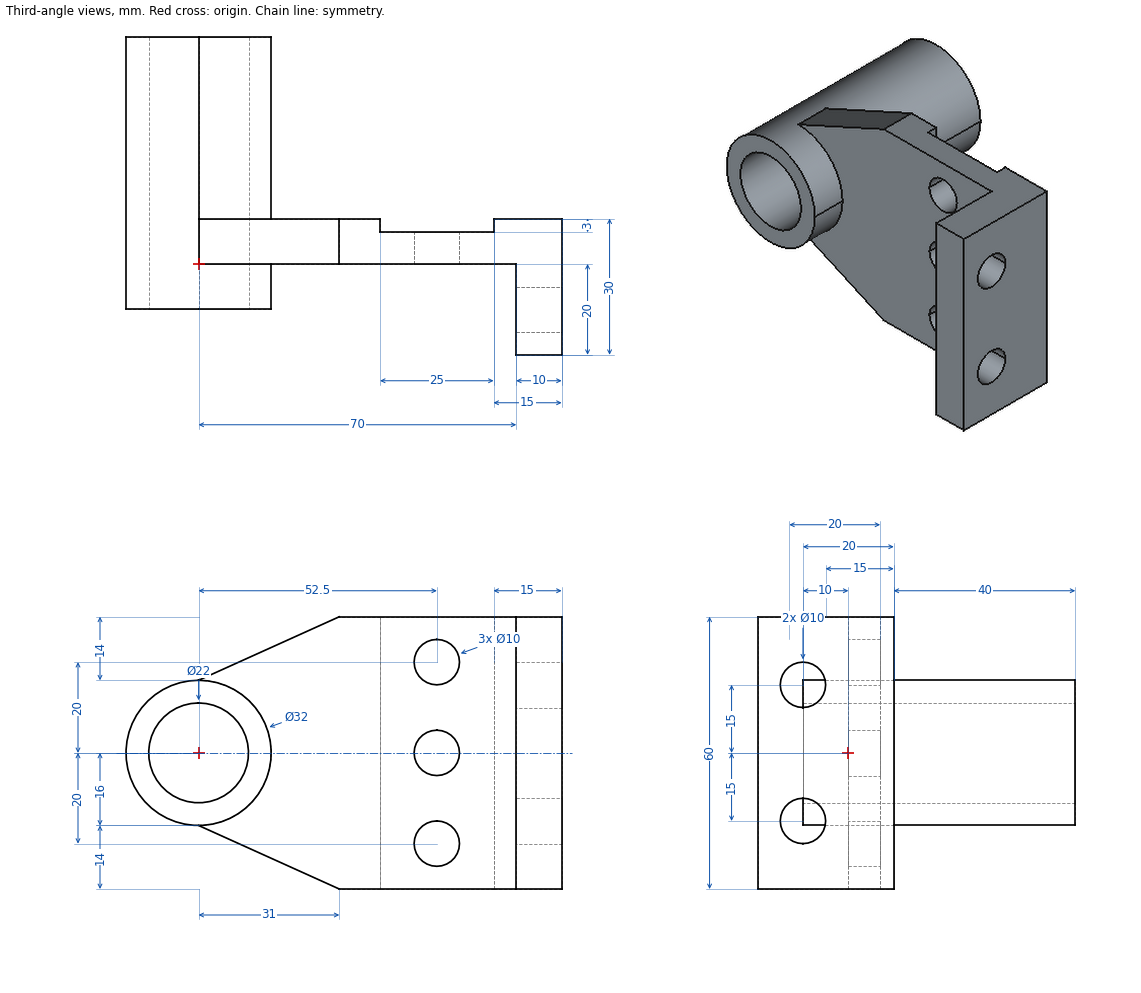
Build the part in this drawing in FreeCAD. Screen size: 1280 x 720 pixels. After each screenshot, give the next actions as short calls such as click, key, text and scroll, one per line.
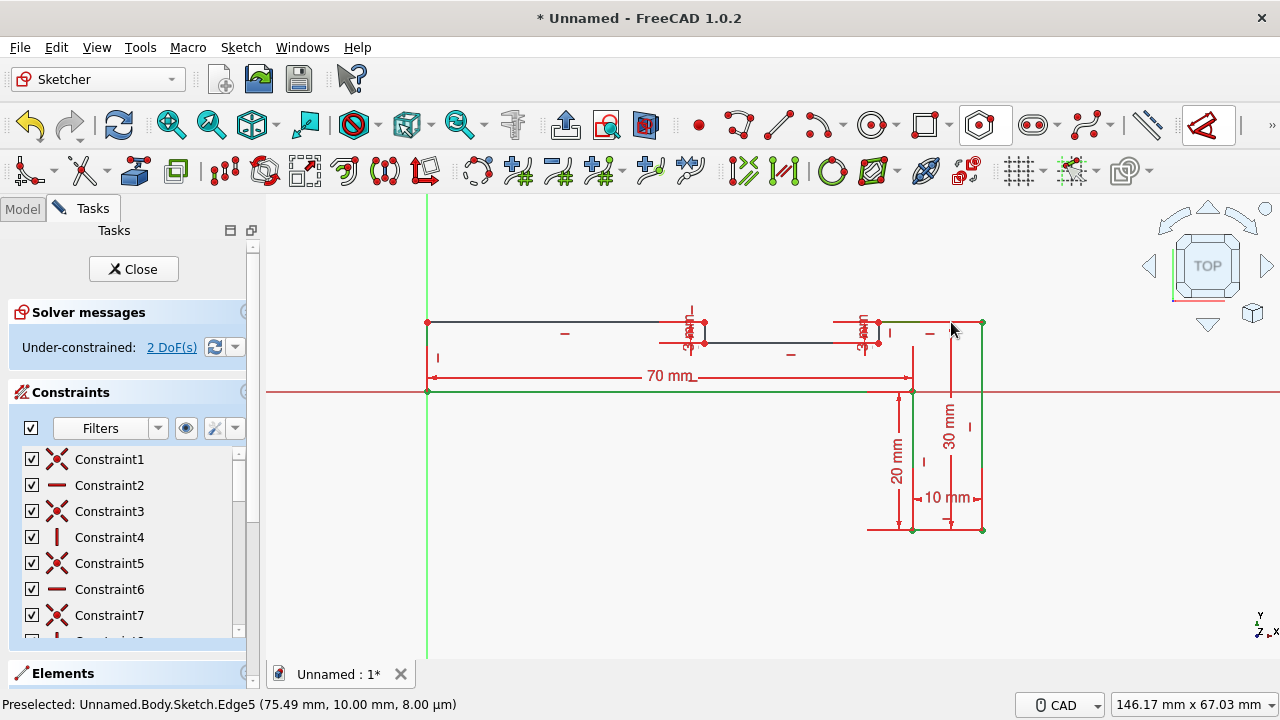
key(l)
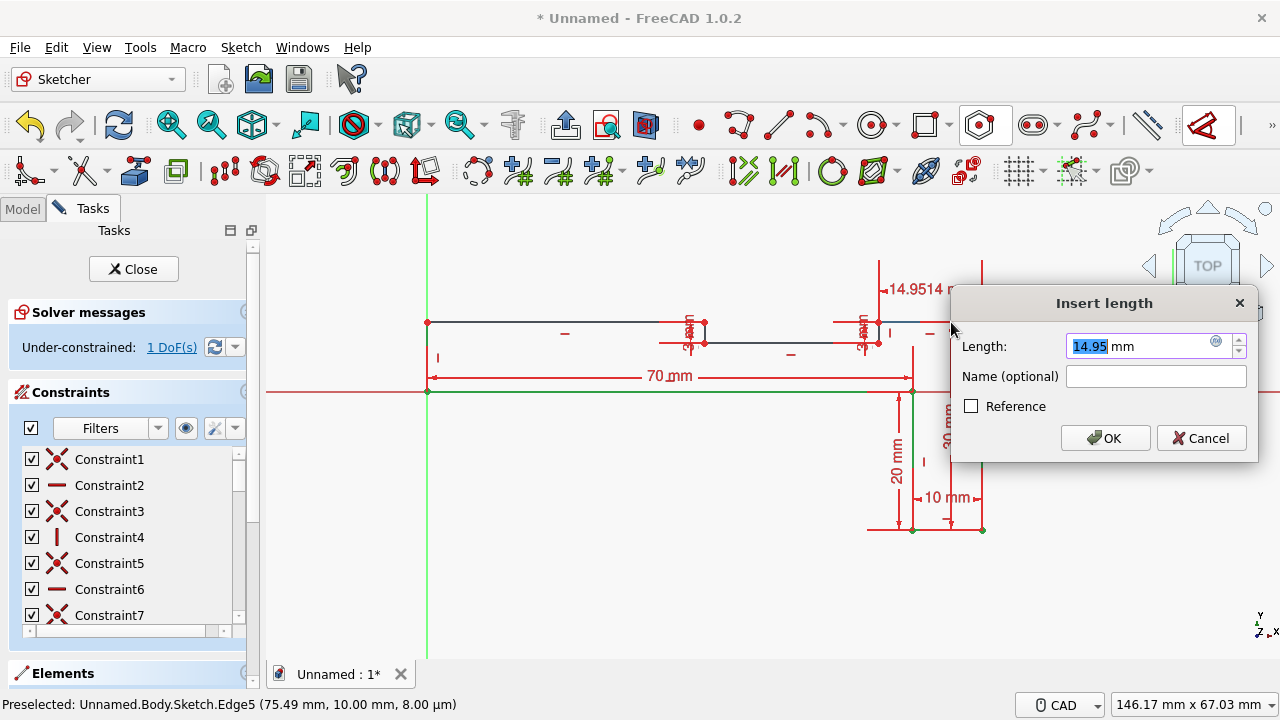
text(15)
key(Return)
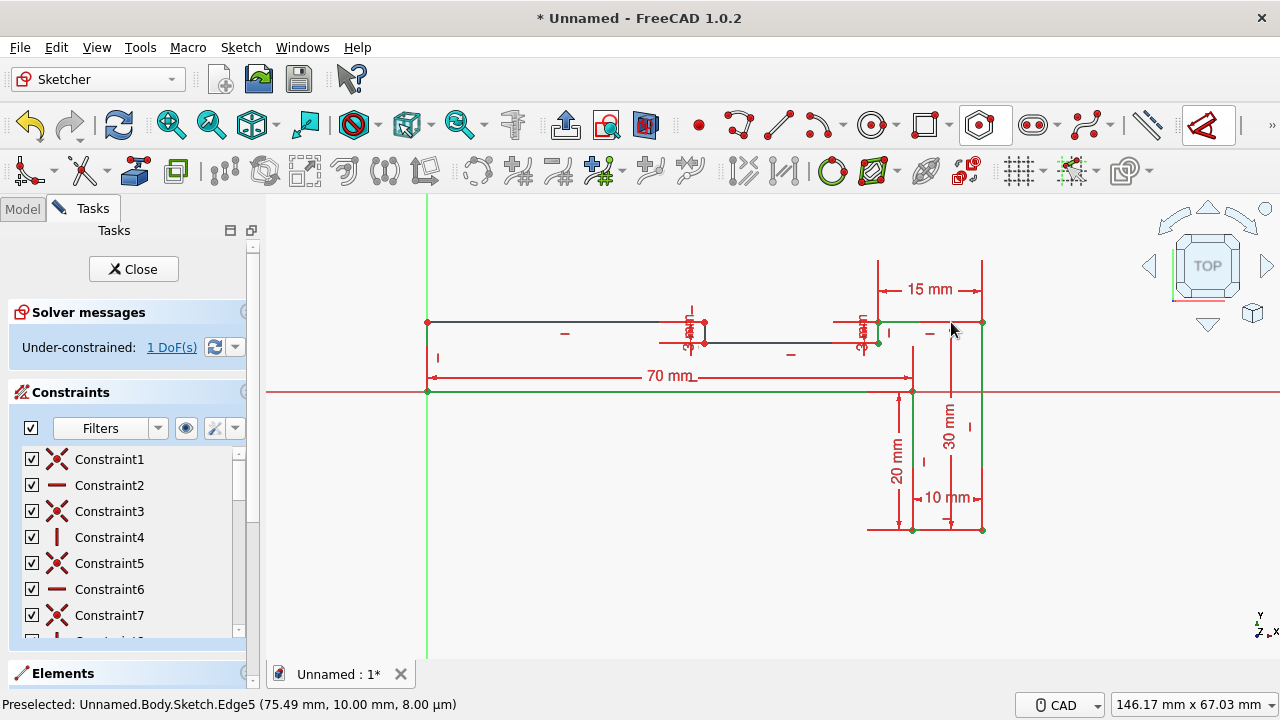
click(826, 343)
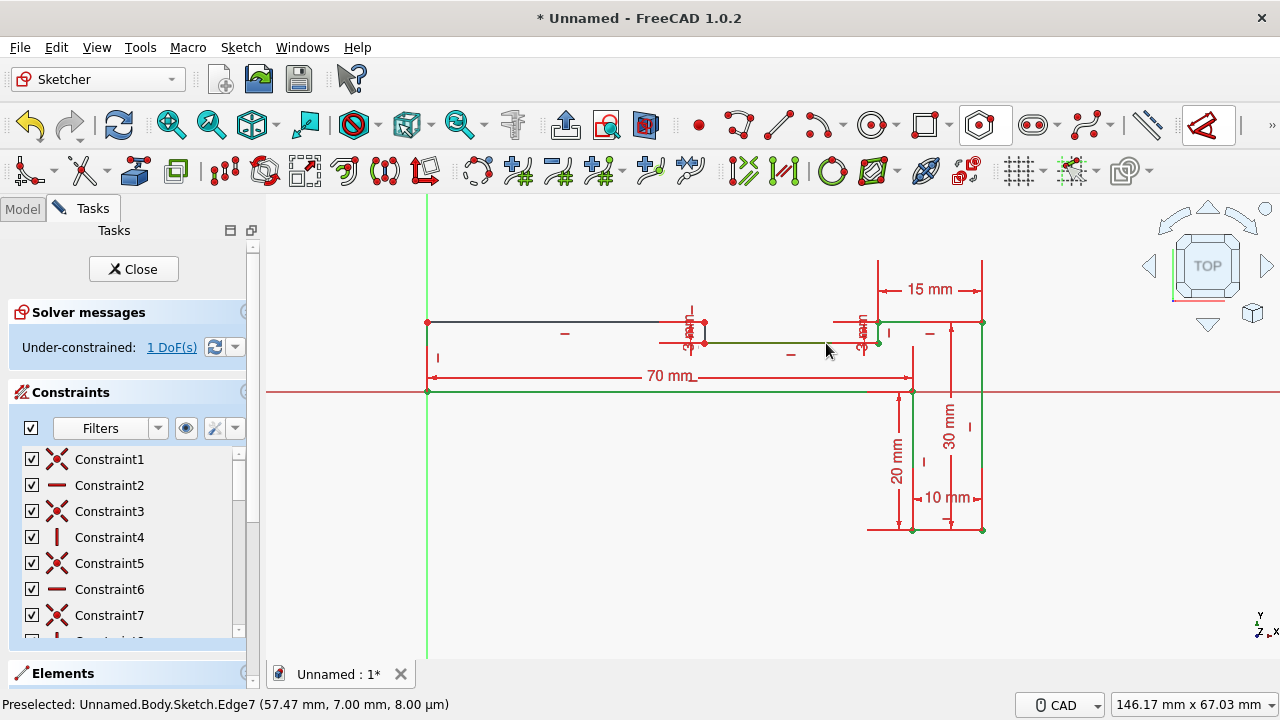
click(1230, 126)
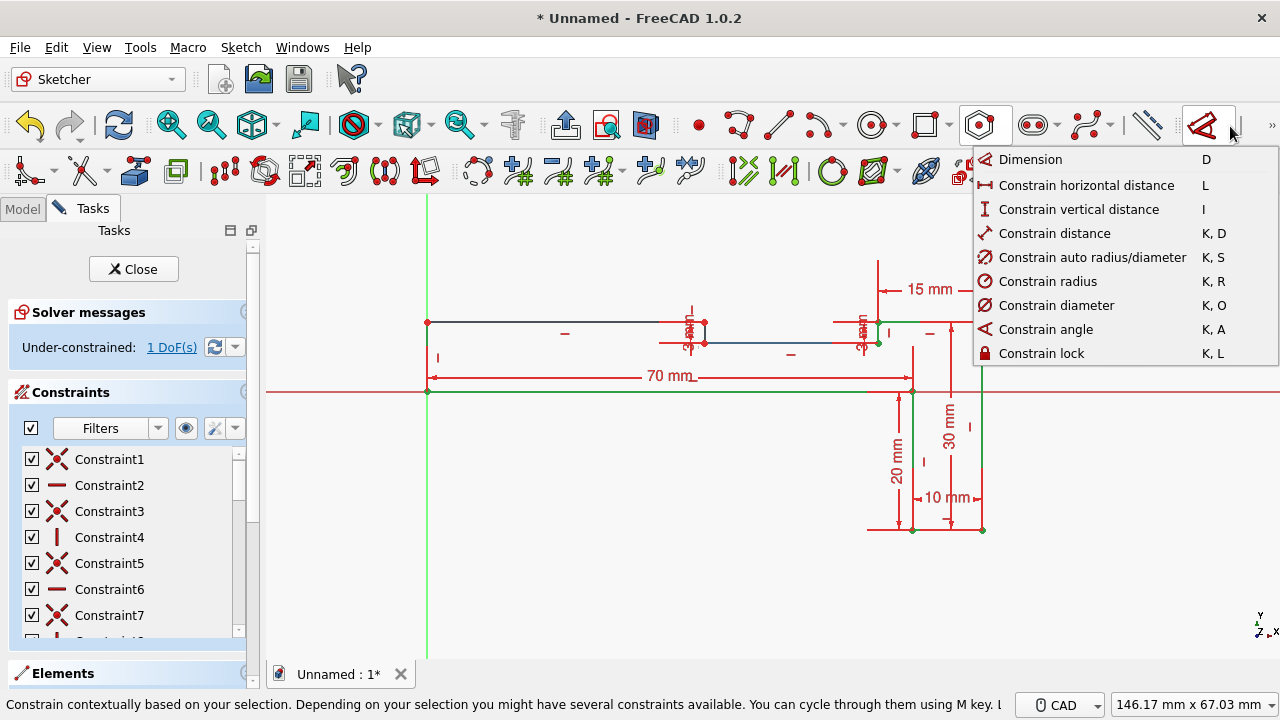
click(1126, 185)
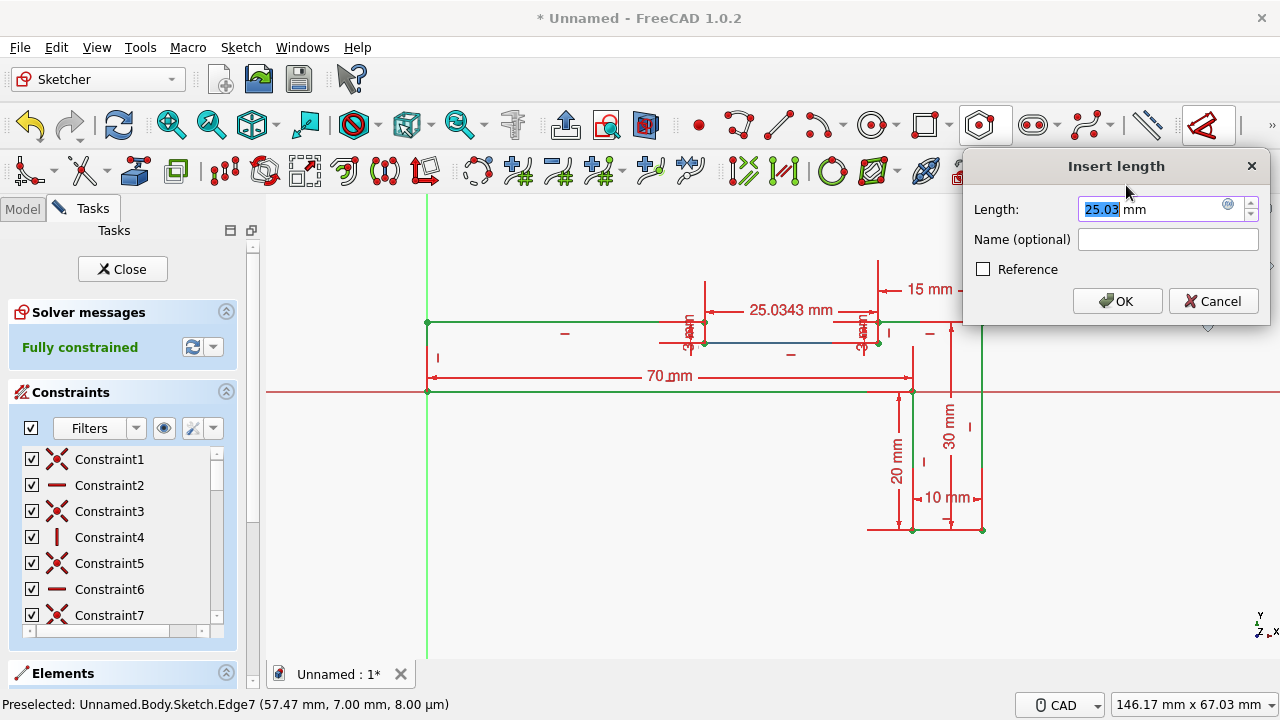
text(25)
key(Return)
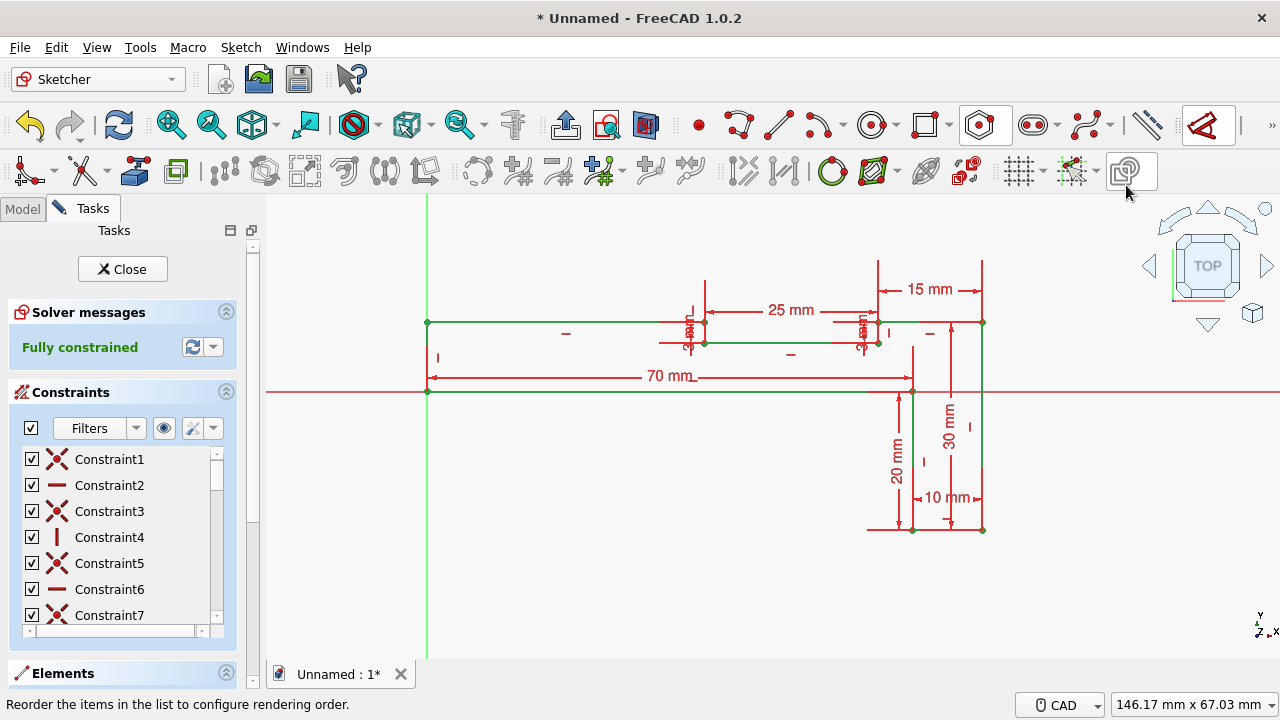
click(123, 269)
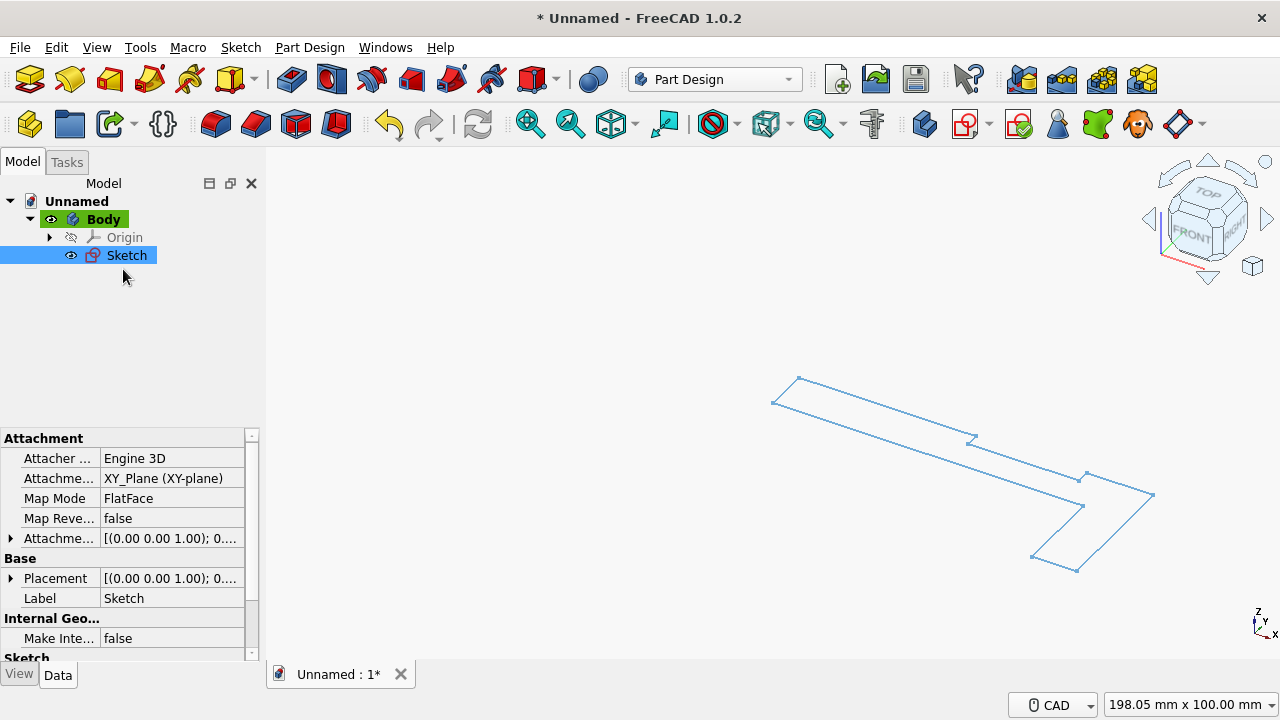
click(30, 80)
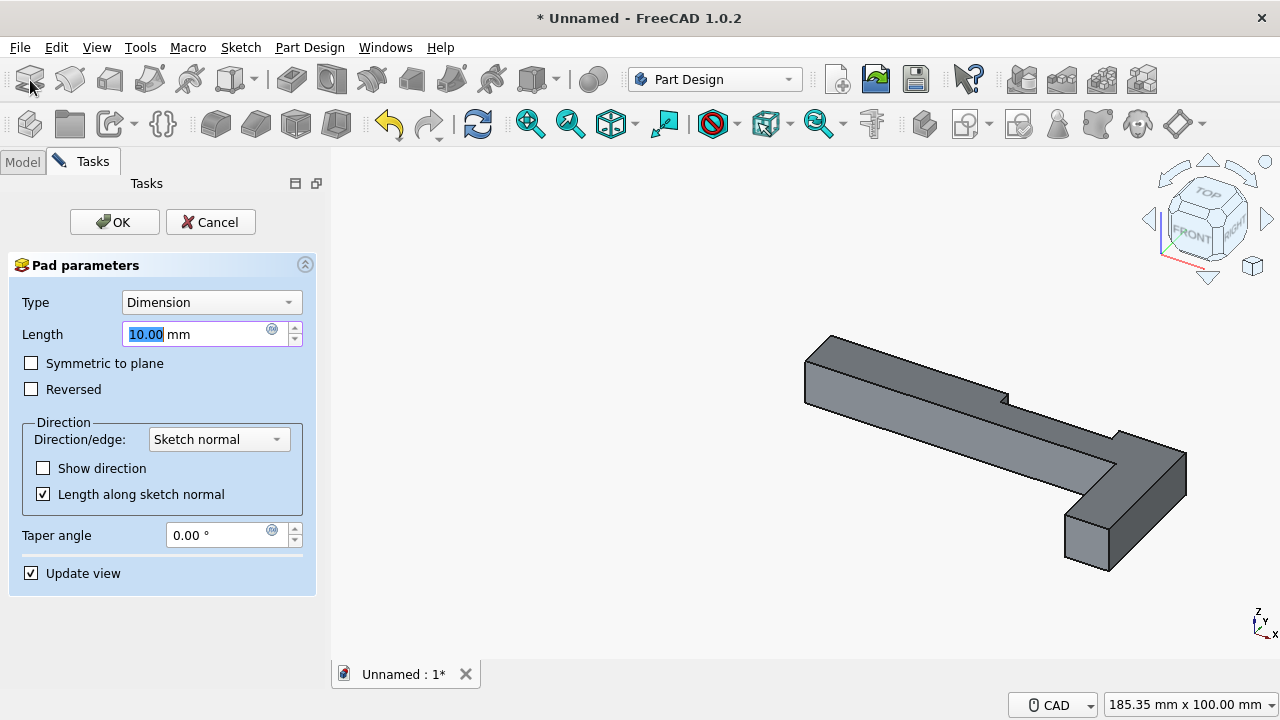
text(60)
key(Tab)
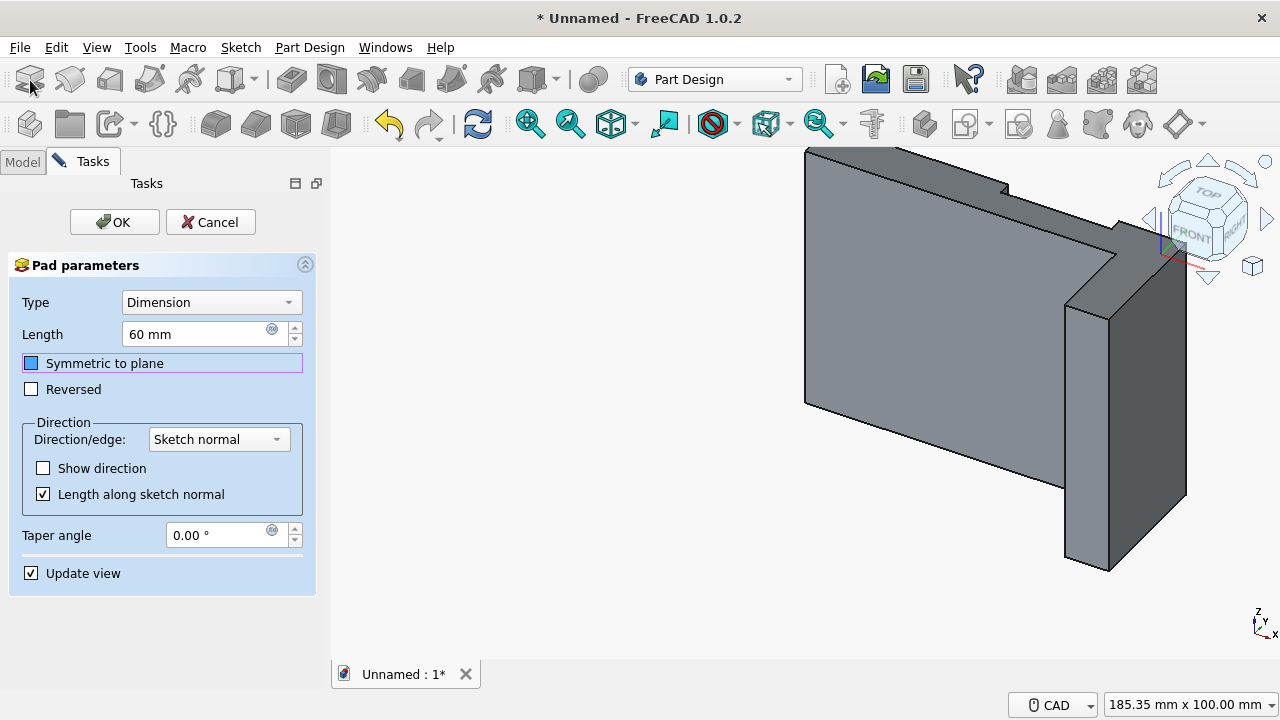
click(30, 363)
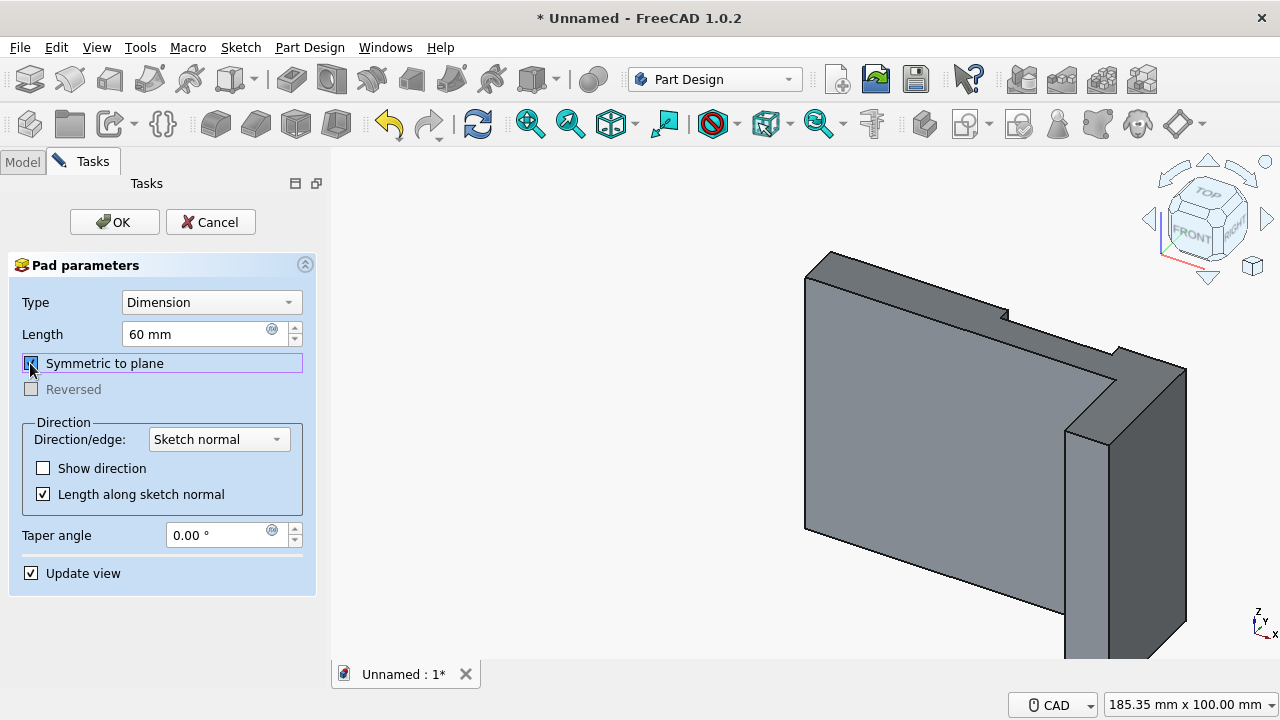
click(115, 222)